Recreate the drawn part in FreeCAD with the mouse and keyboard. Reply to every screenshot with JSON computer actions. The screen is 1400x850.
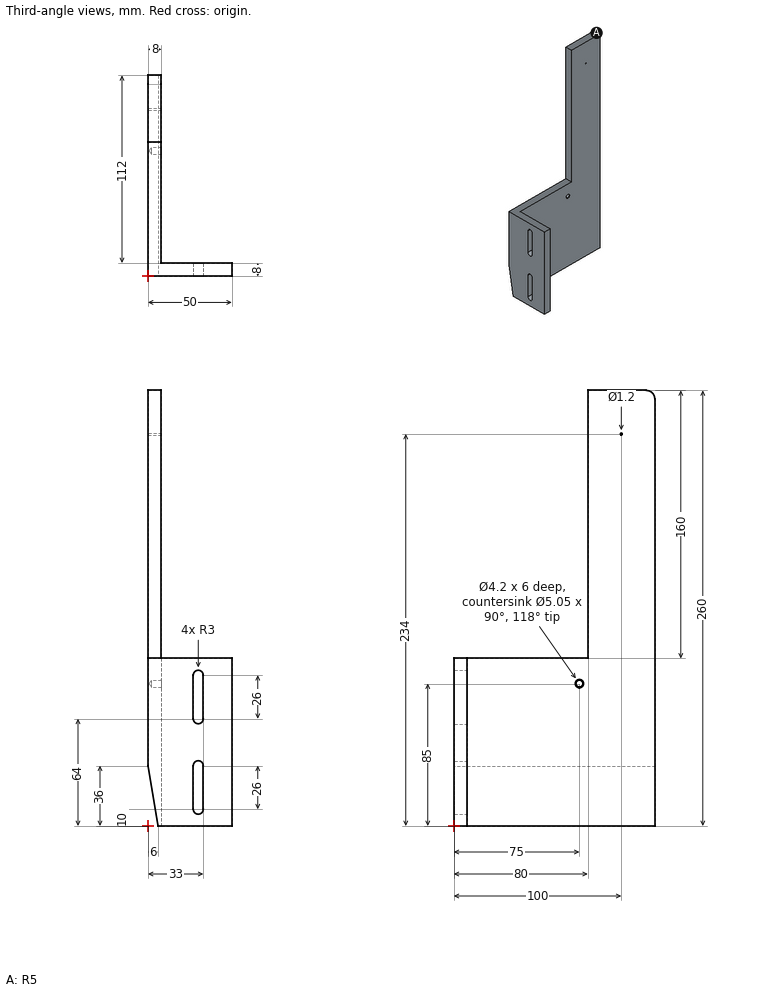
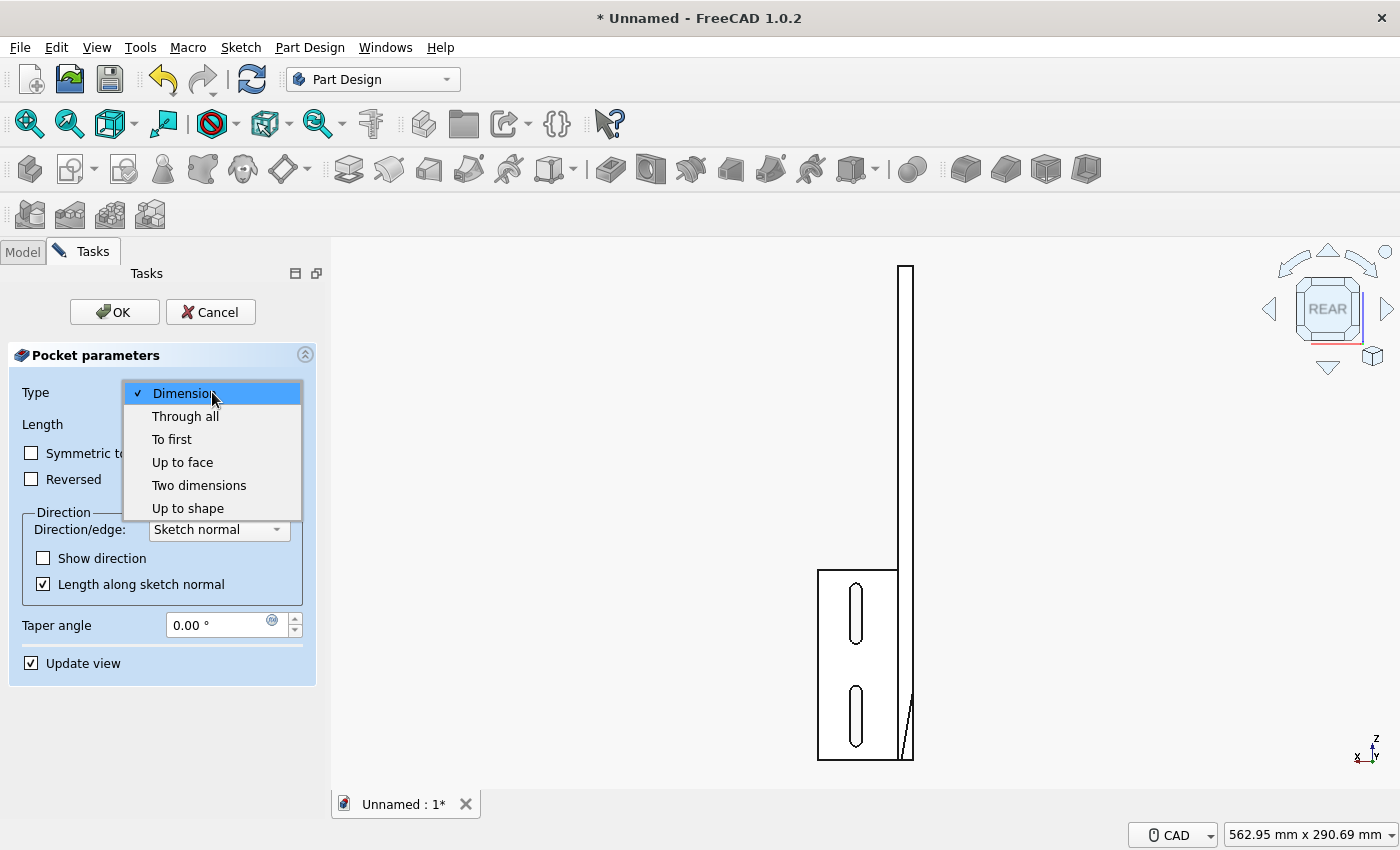
{"action": "left_click", "coordinate": [212, 416]}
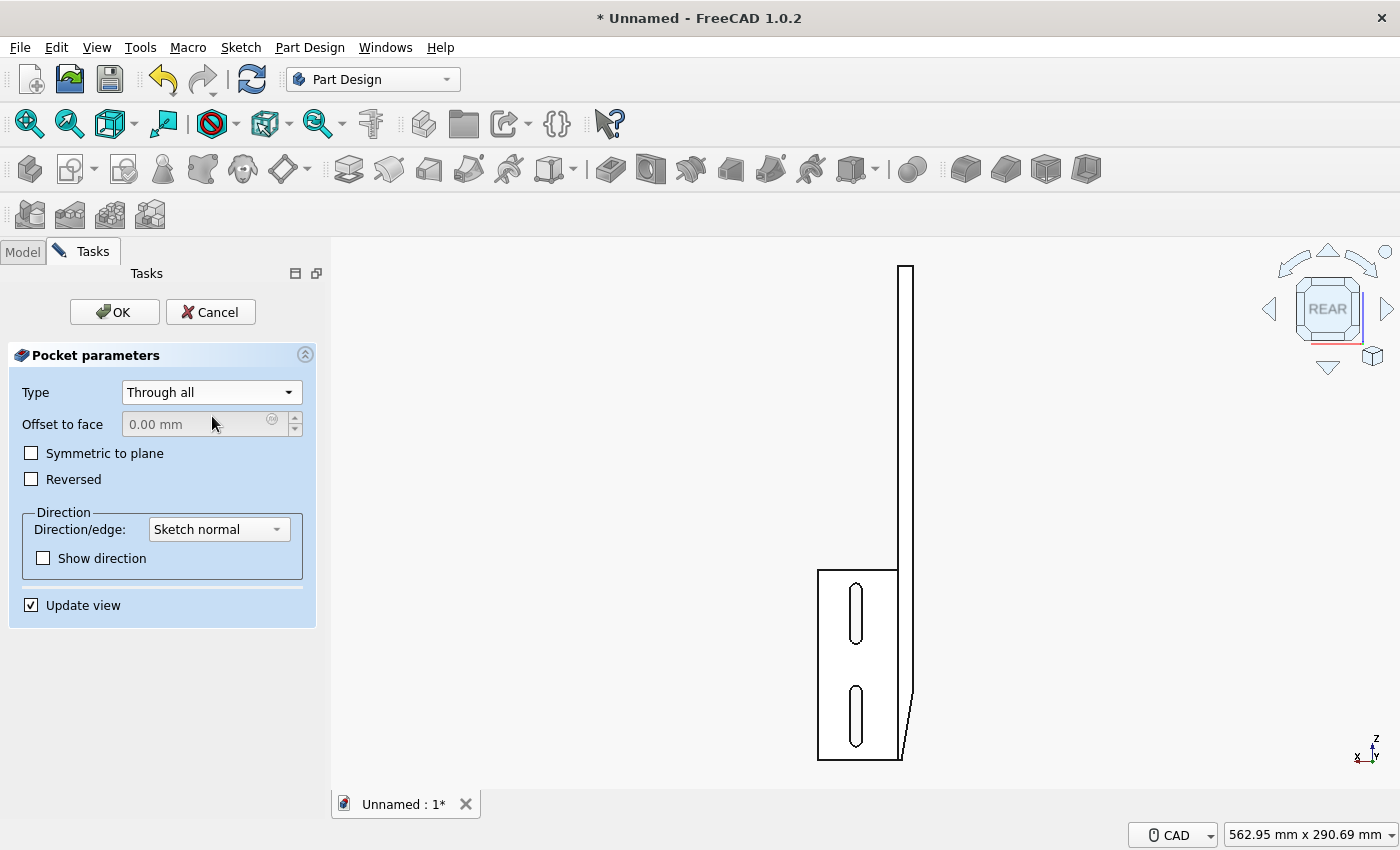
{"action": "left_click", "coordinate": [115, 312]}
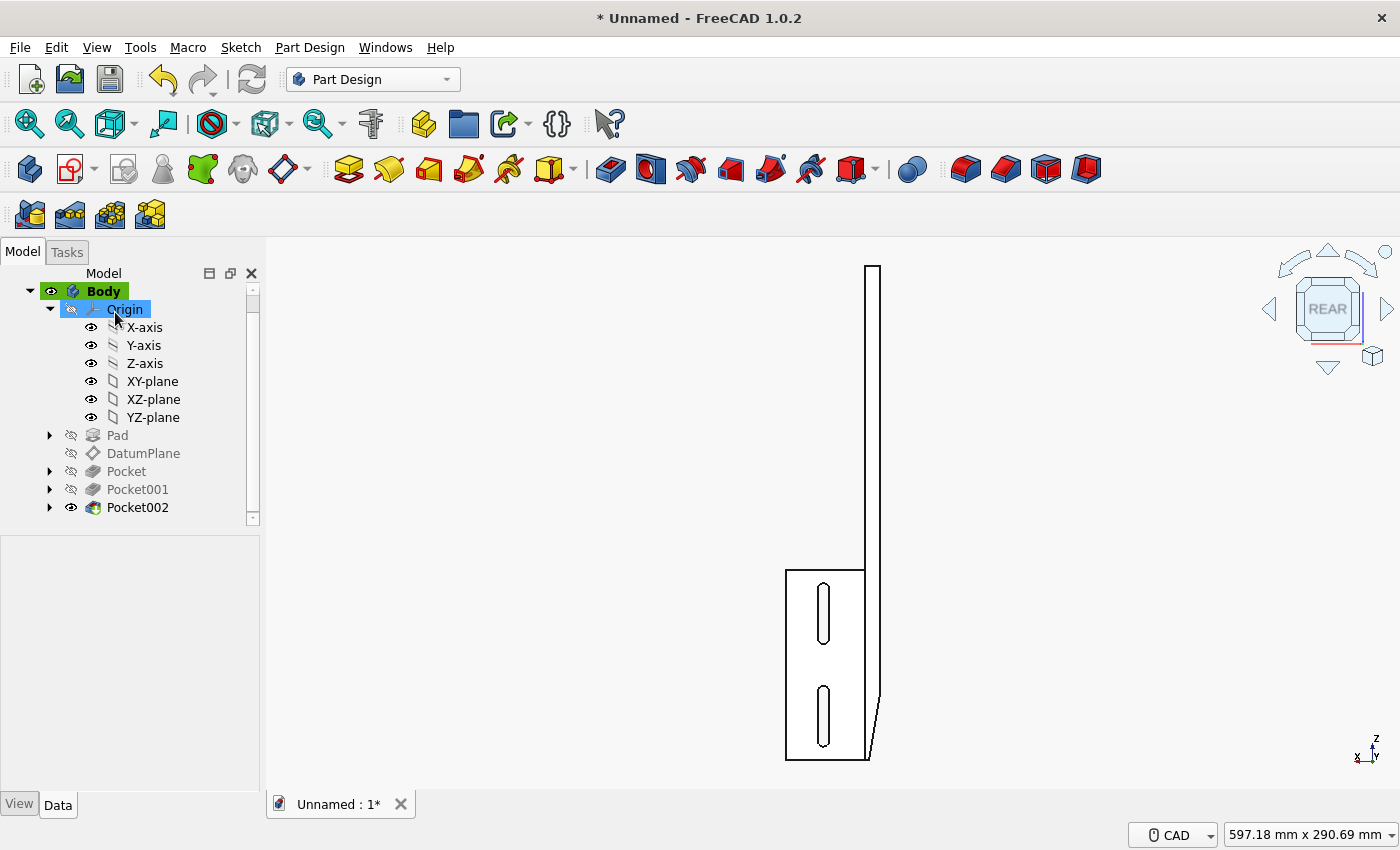
{"action": "key", "text": "0"}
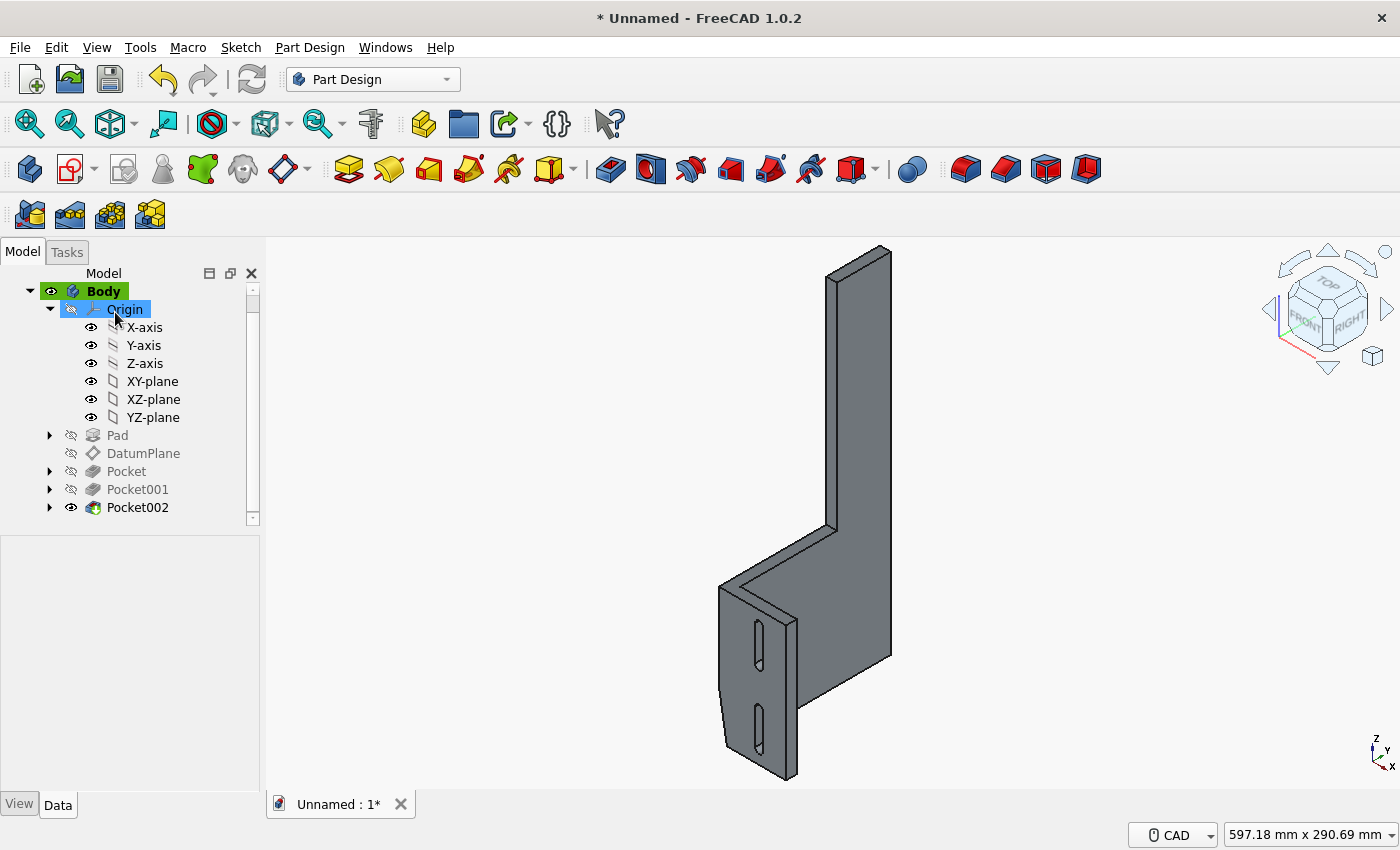
{"action": "left_click", "coordinate": [816, 611]}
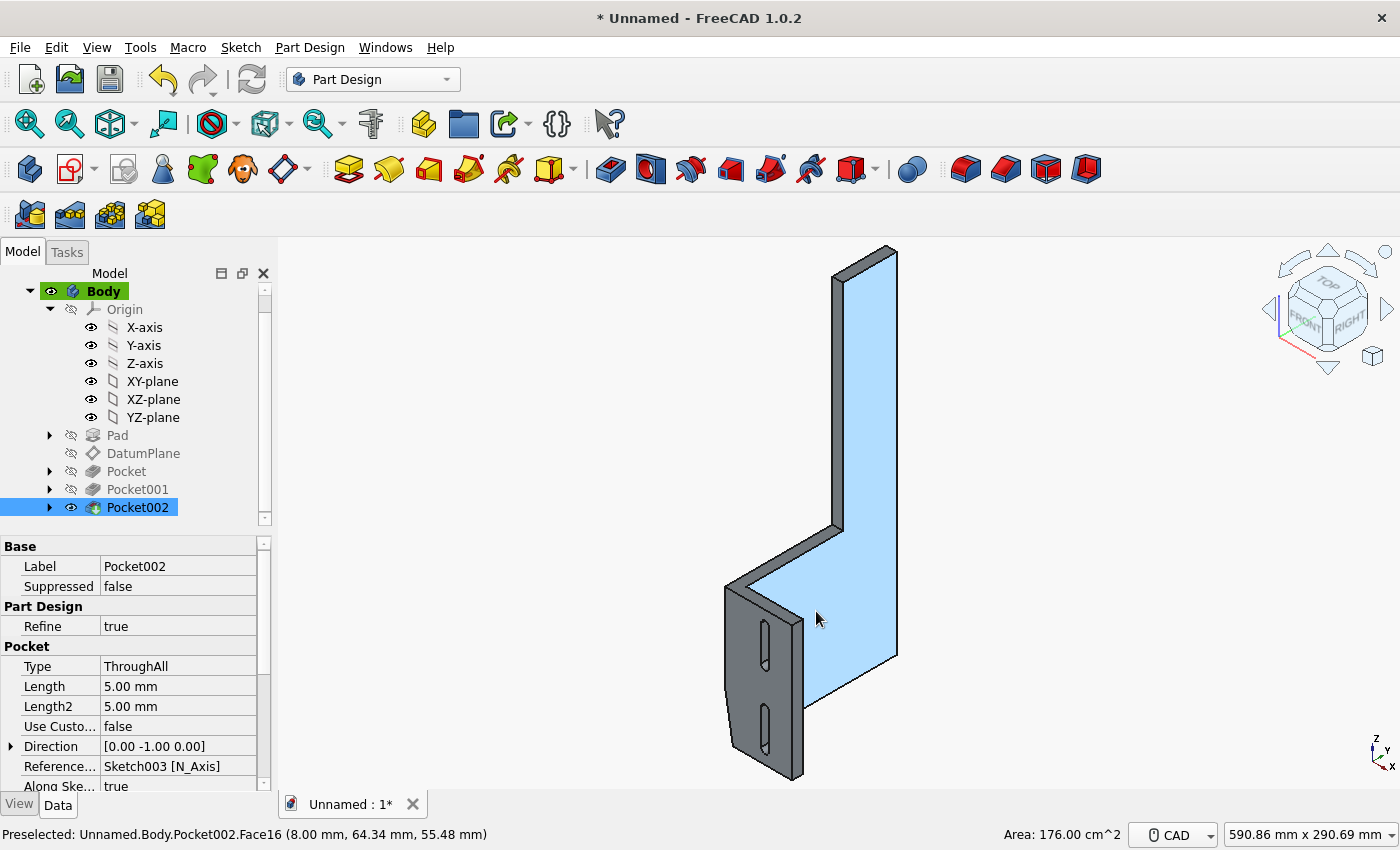
{"action": "left_click", "coordinate": [70, 170]}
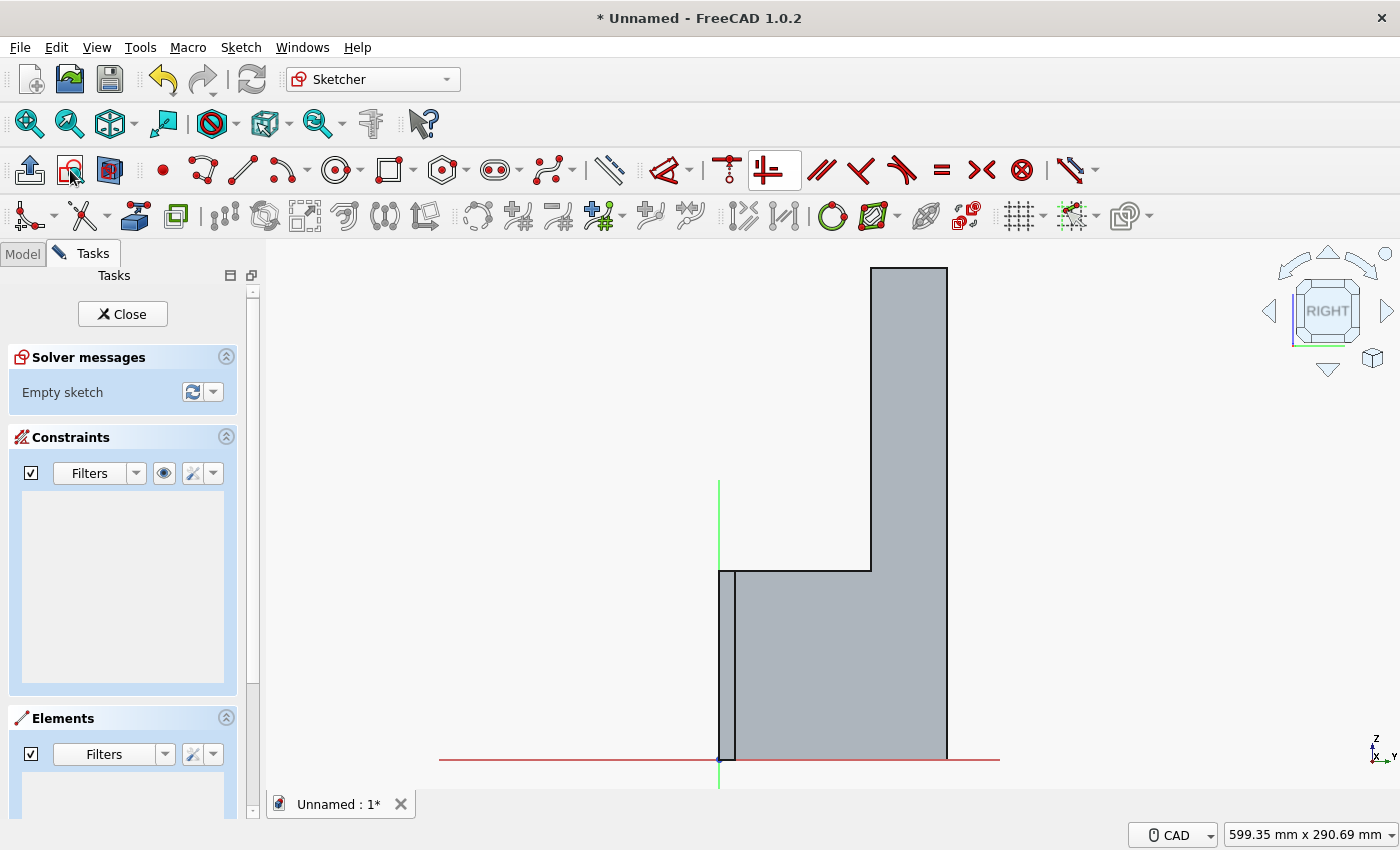
{"action": "scroll", "coordinate": [866, 604], "scroll_direction": "up", "scroll_amount": 15}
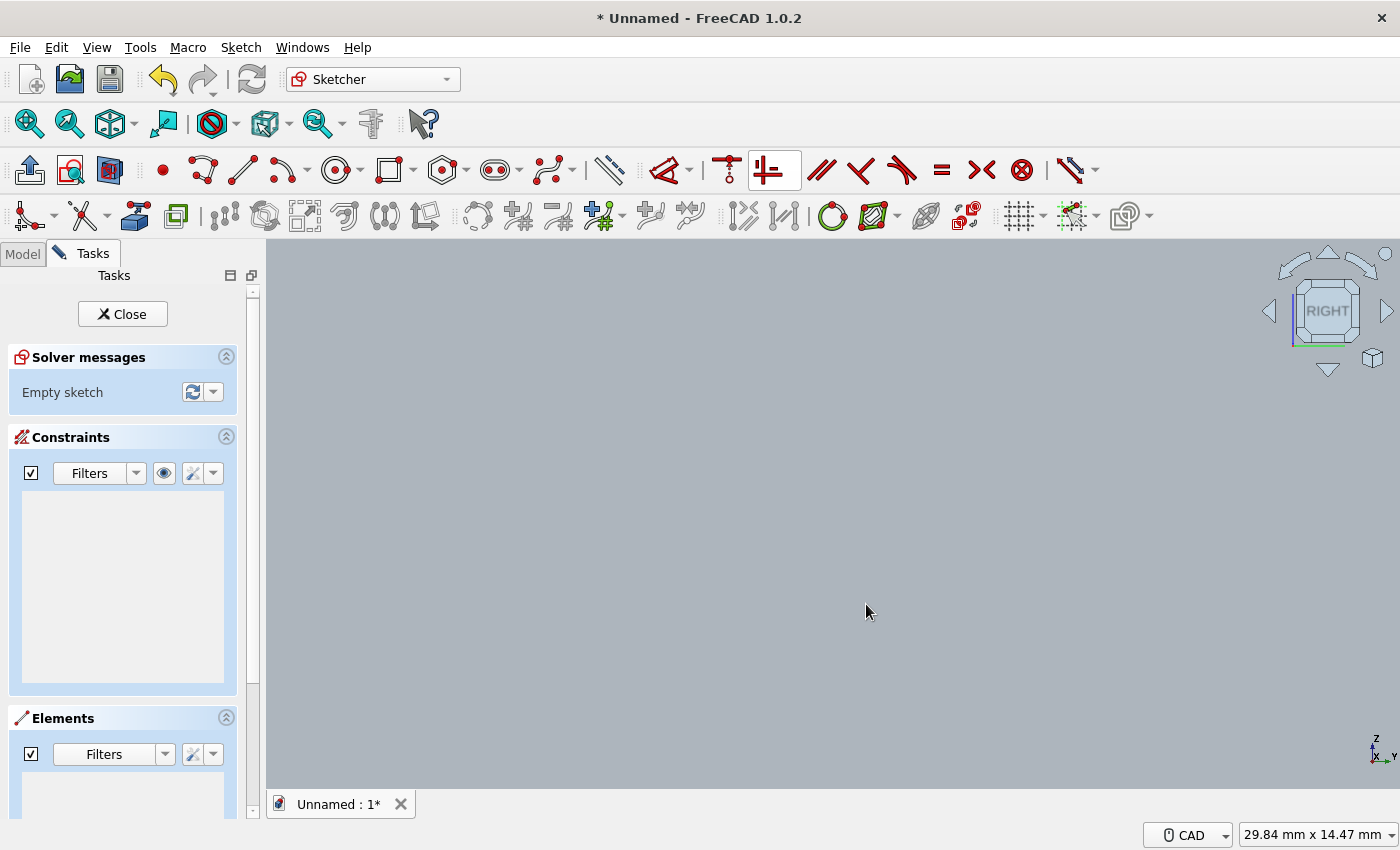
{"action": "scroll", "coordinate": [762, 477], "scroll_direction": "up", "scroll_amount": 4}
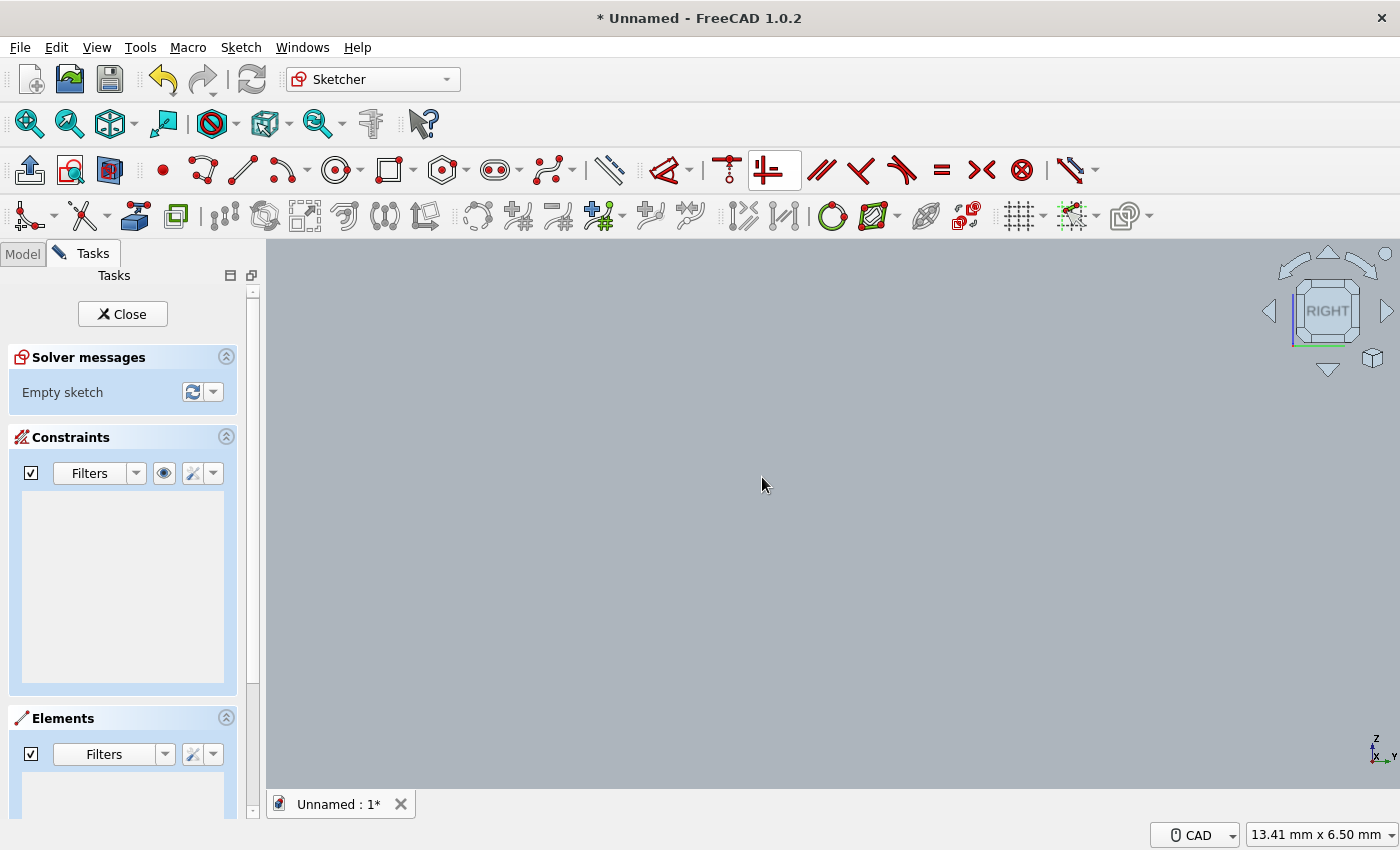
{"action": "left_click", "coordinate": [336, 170]}